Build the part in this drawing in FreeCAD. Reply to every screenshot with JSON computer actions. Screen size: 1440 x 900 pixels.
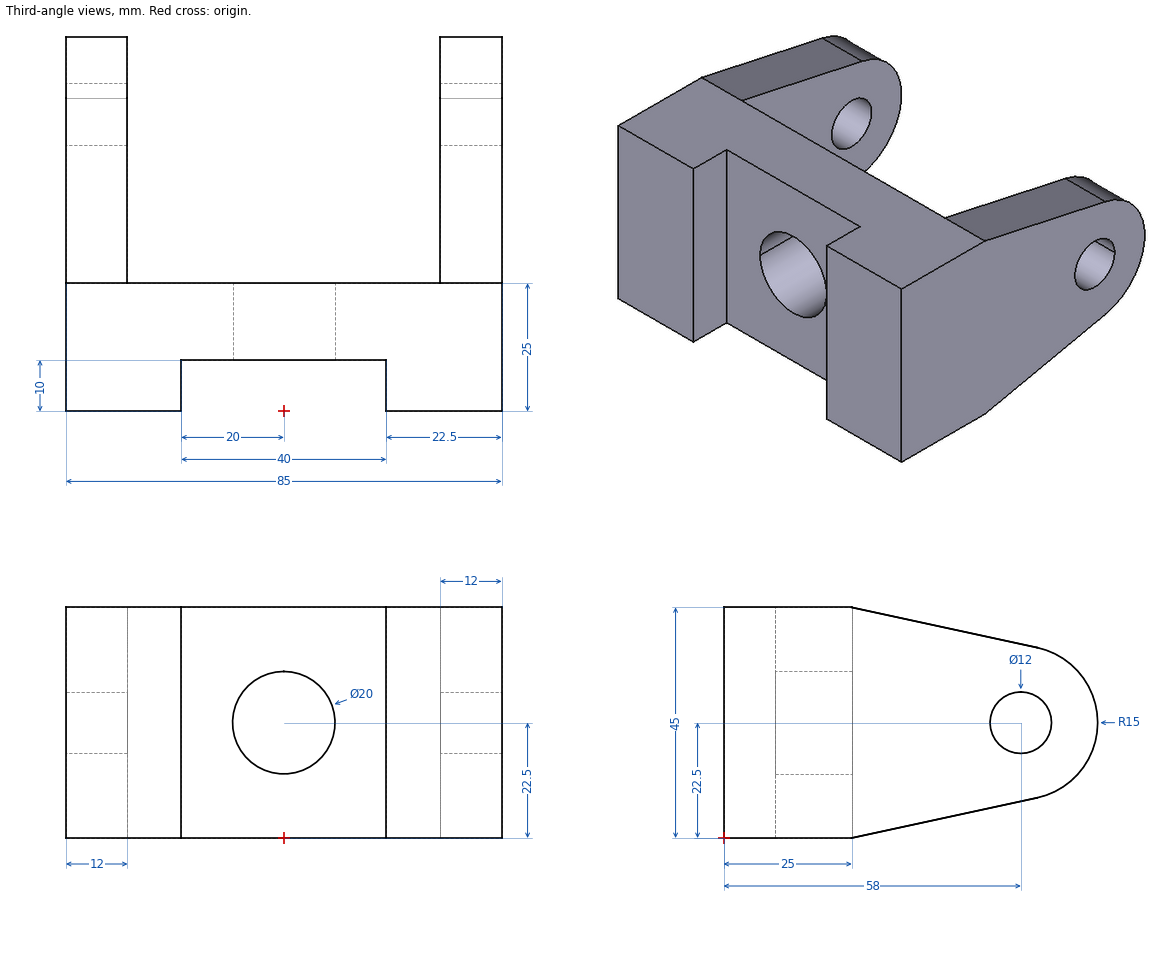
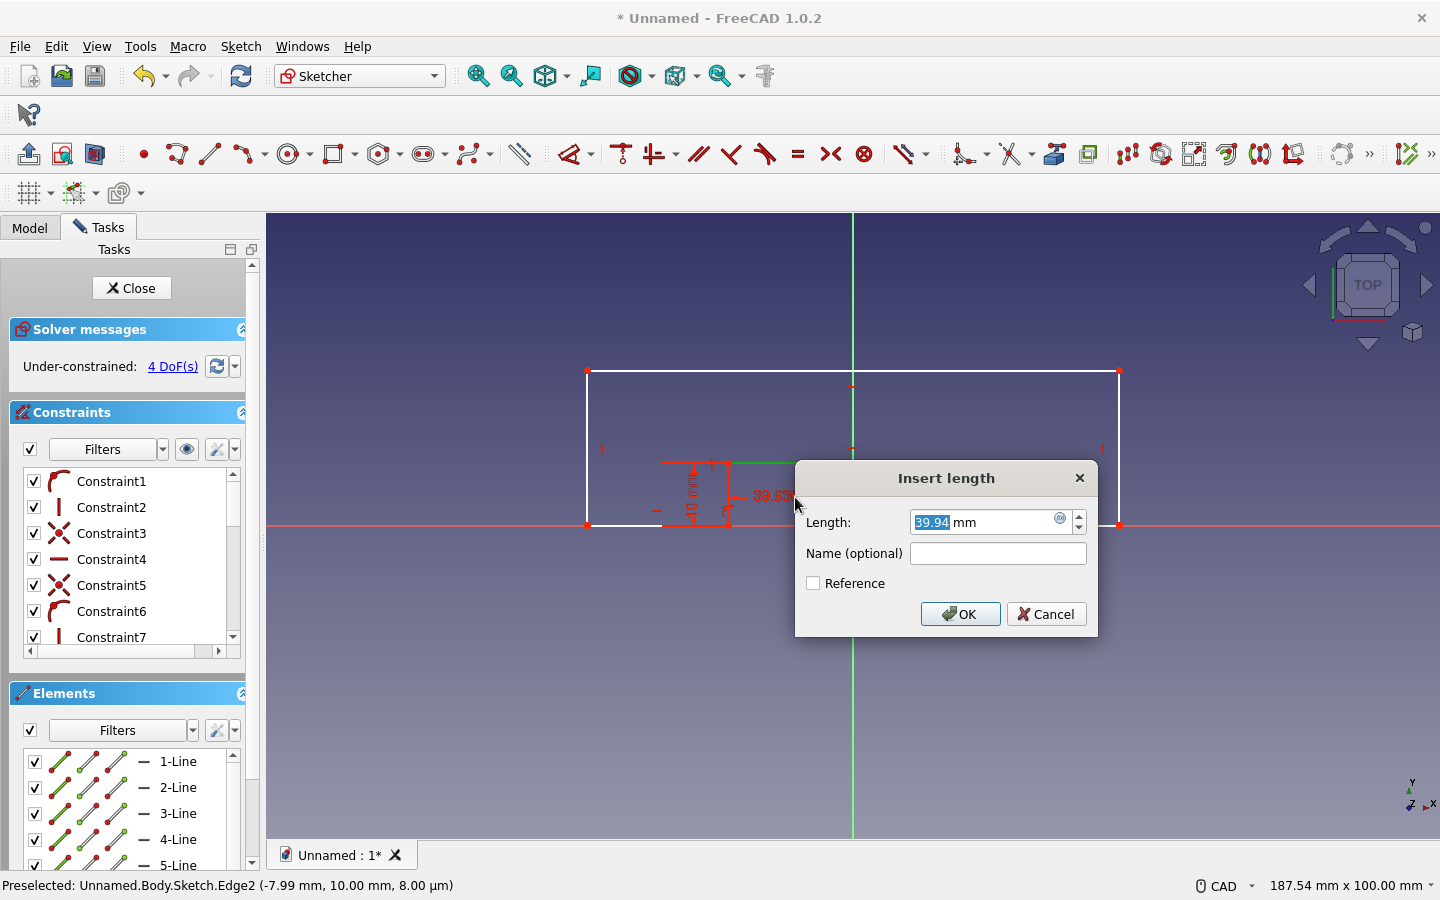
{"action": "type", "text": "40"}
{"action": "key", "text": "Return"}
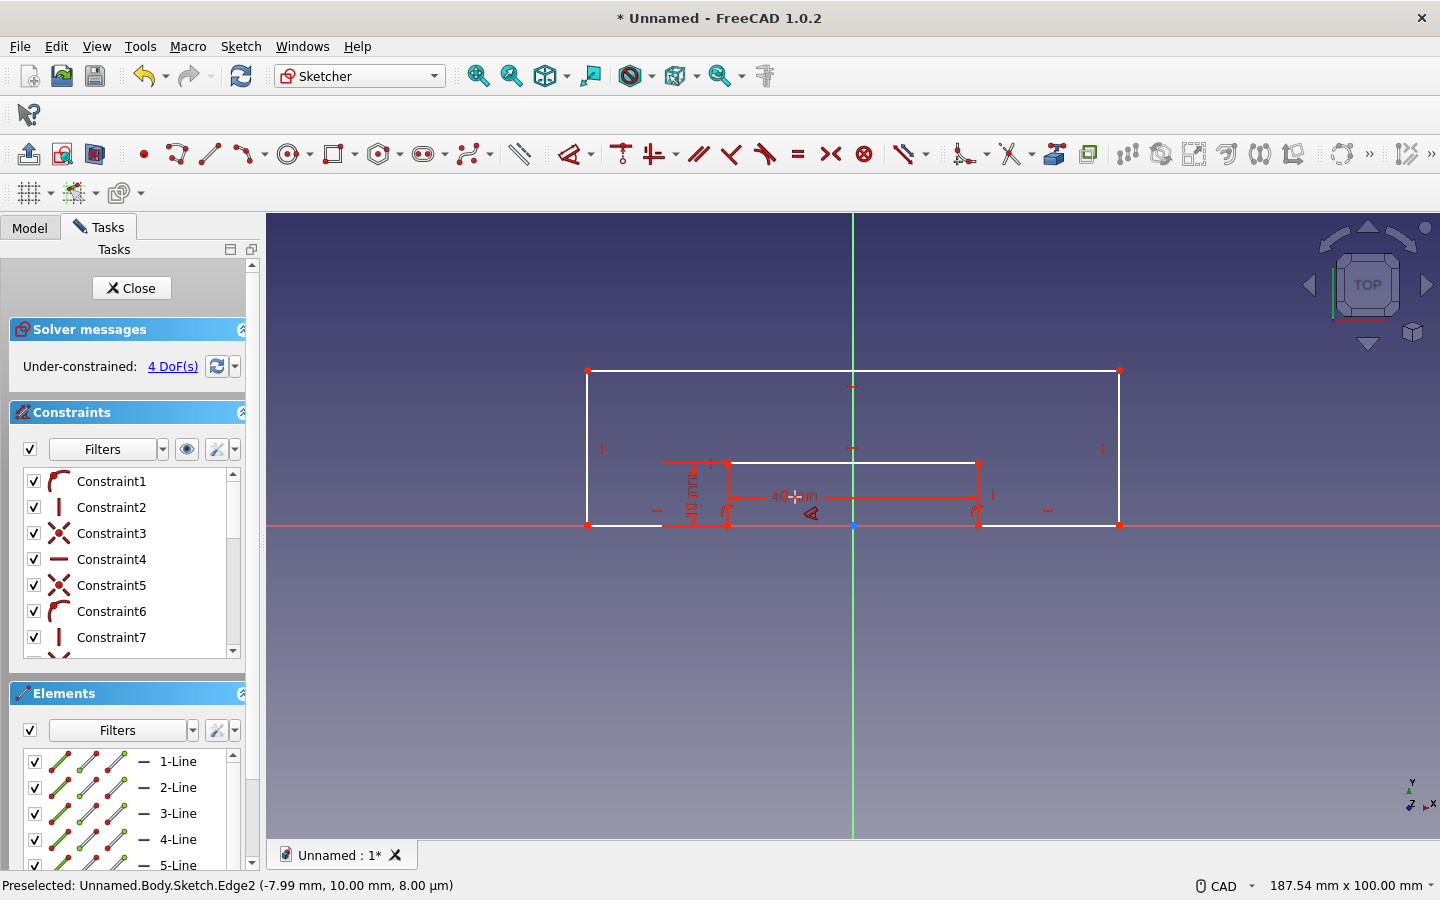
{"action": "left_click", "coordinate": [1119, 479]}
{"action": "left_click", "coordinate": [1153, 448]}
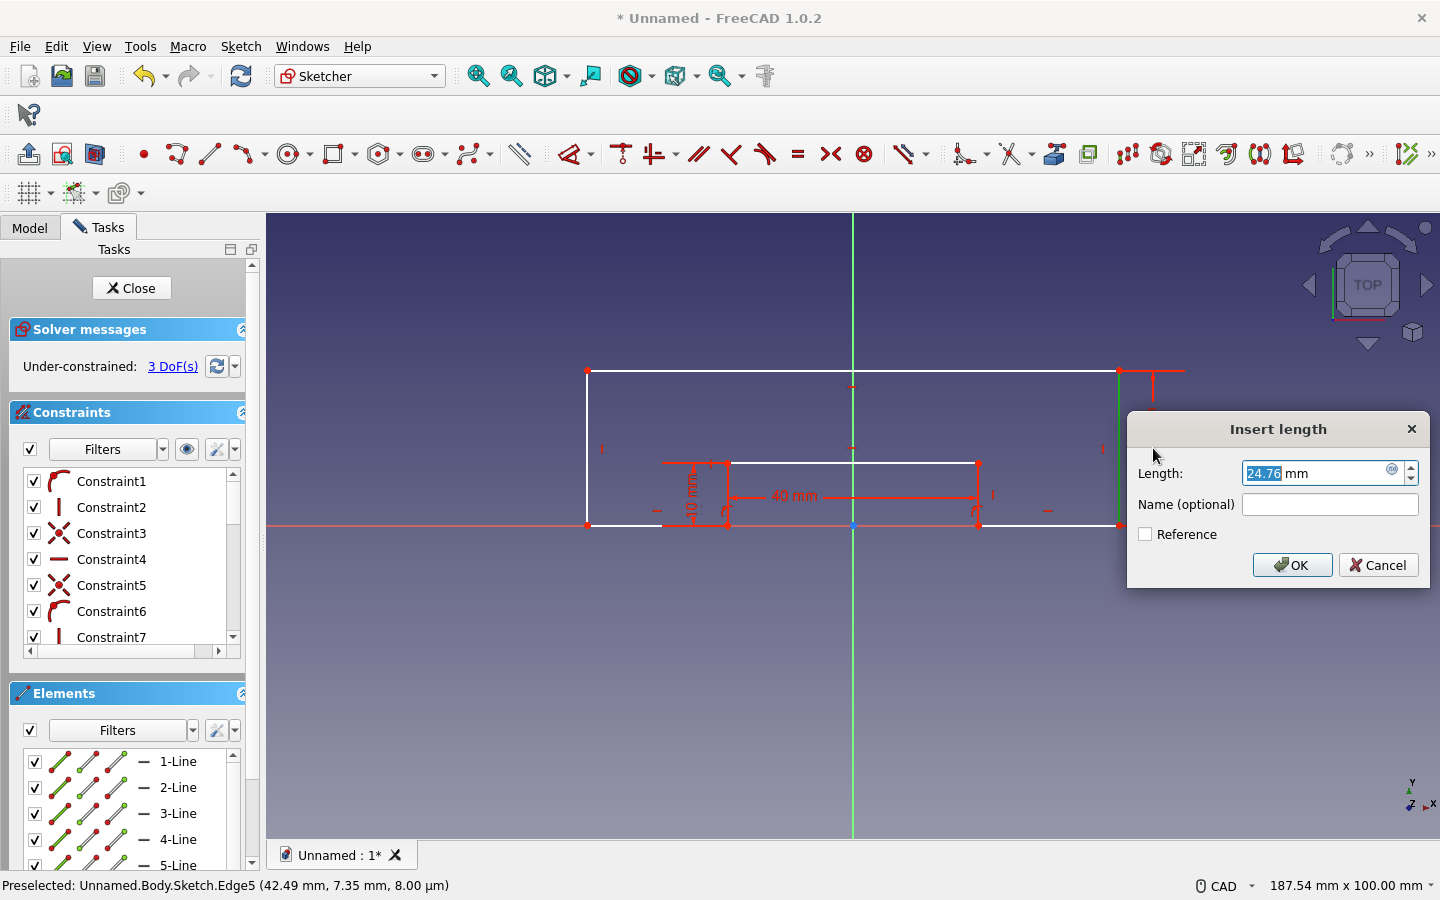
{"action": "type", "text": "25"}
{"action": "key", "text": "Return"}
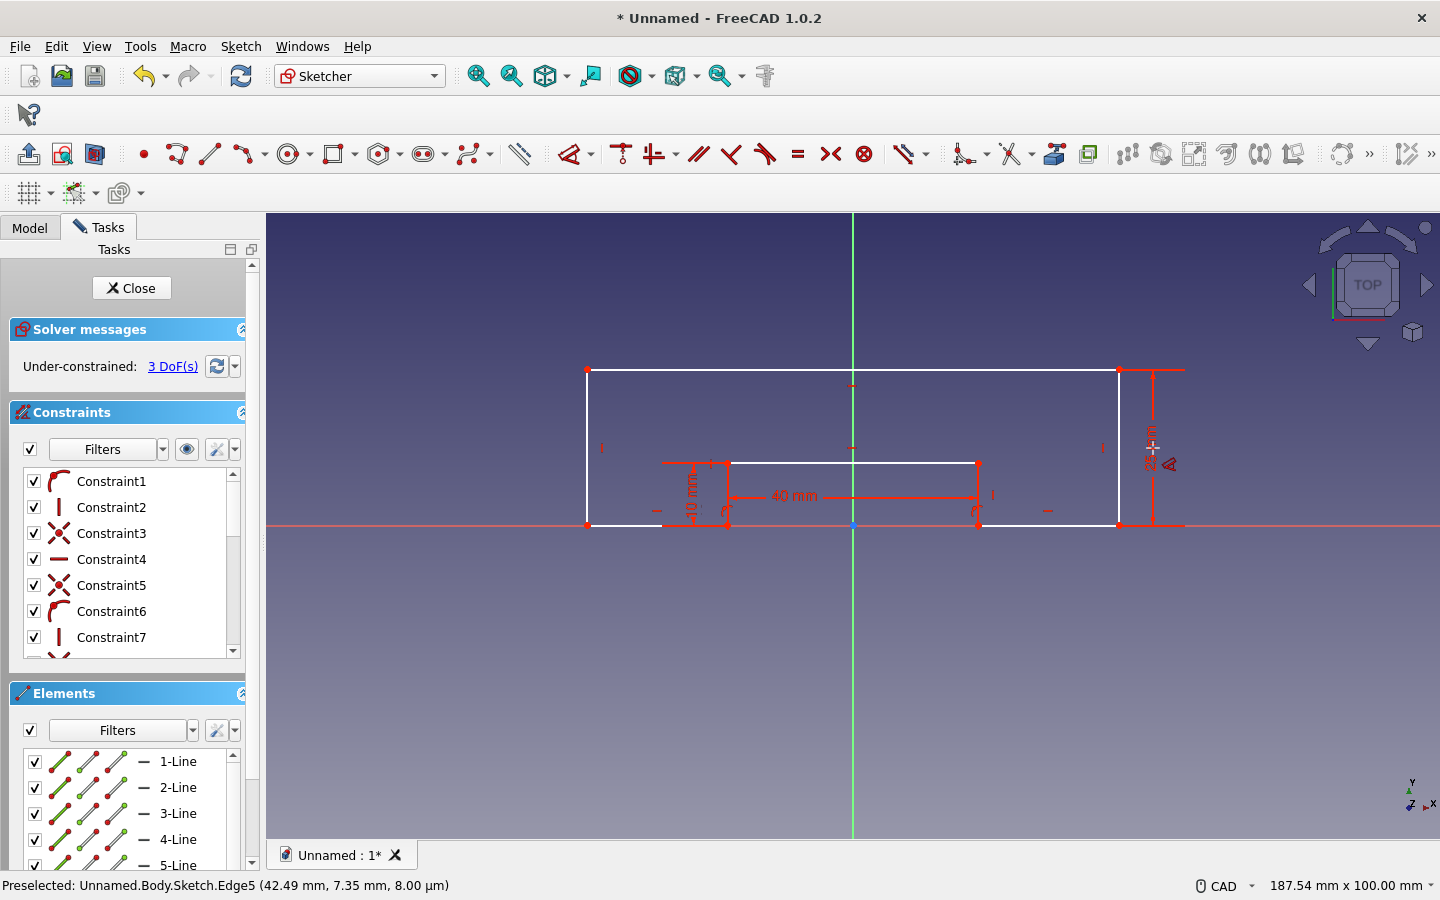
{"action": "left_click", "coordinate": [959, 370]}
{"action": "left_click", "coordinate": [731, 336]}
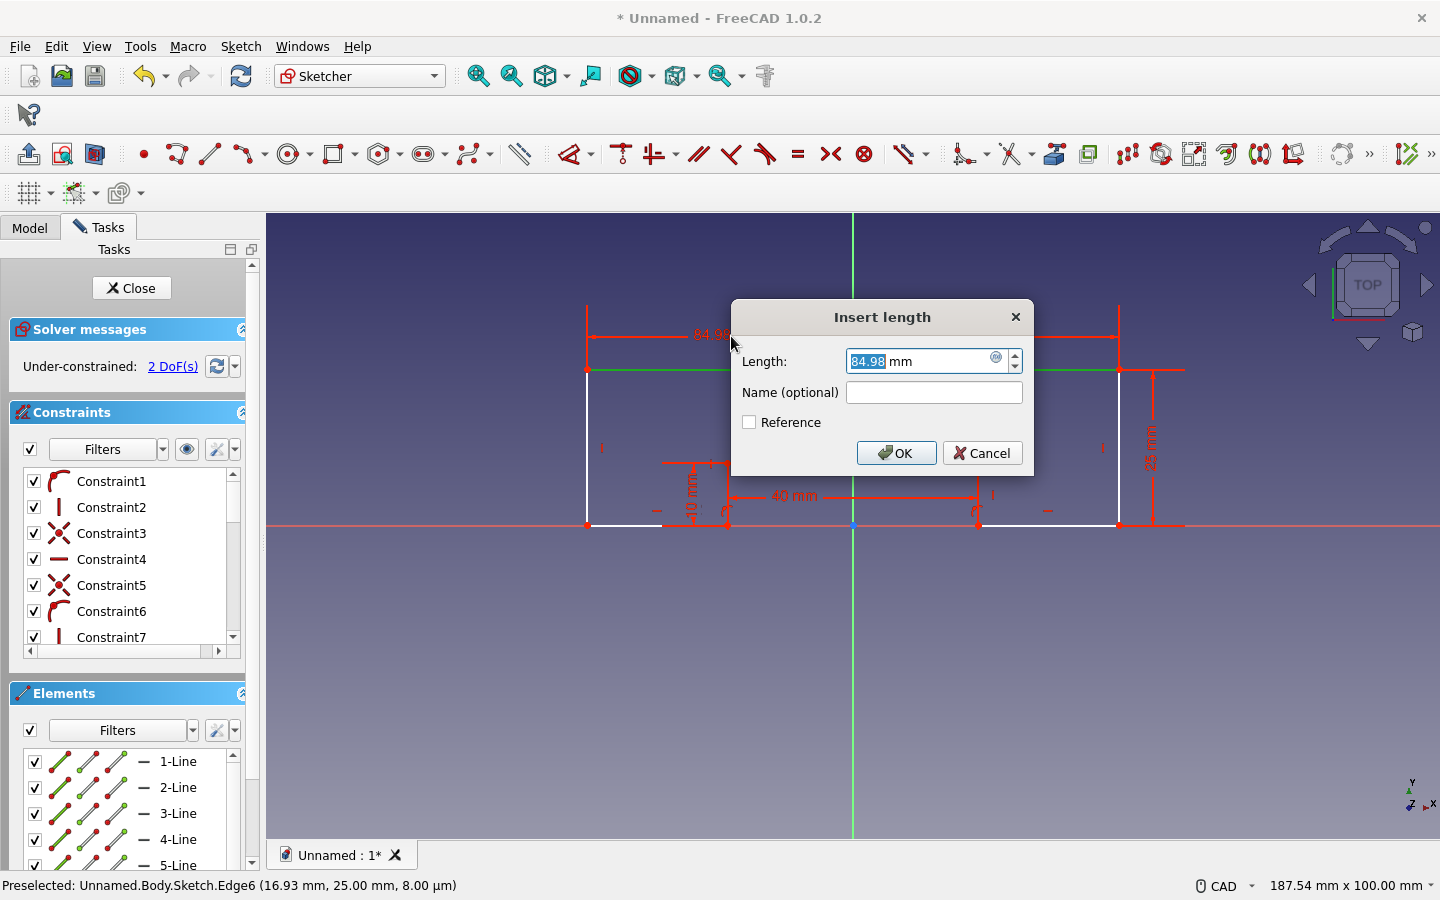
{"action": "type", "text": "85"}
{"action": "key", "text": "Return"}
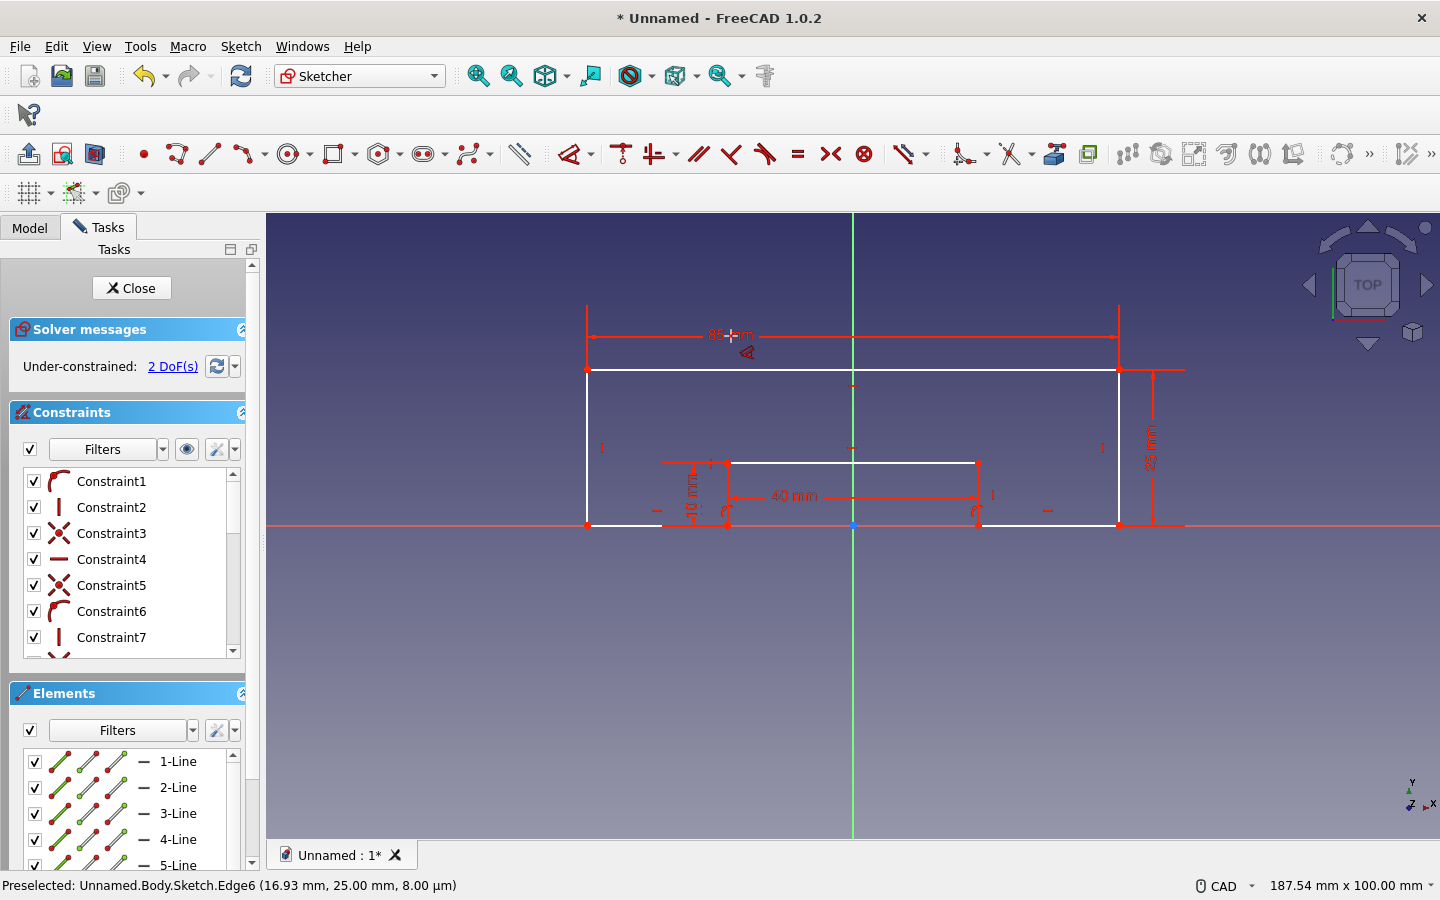
{"action": "left_click", "coordinate": [728, 526]}
{"action": "left_click", "coordinate": [790, 560]}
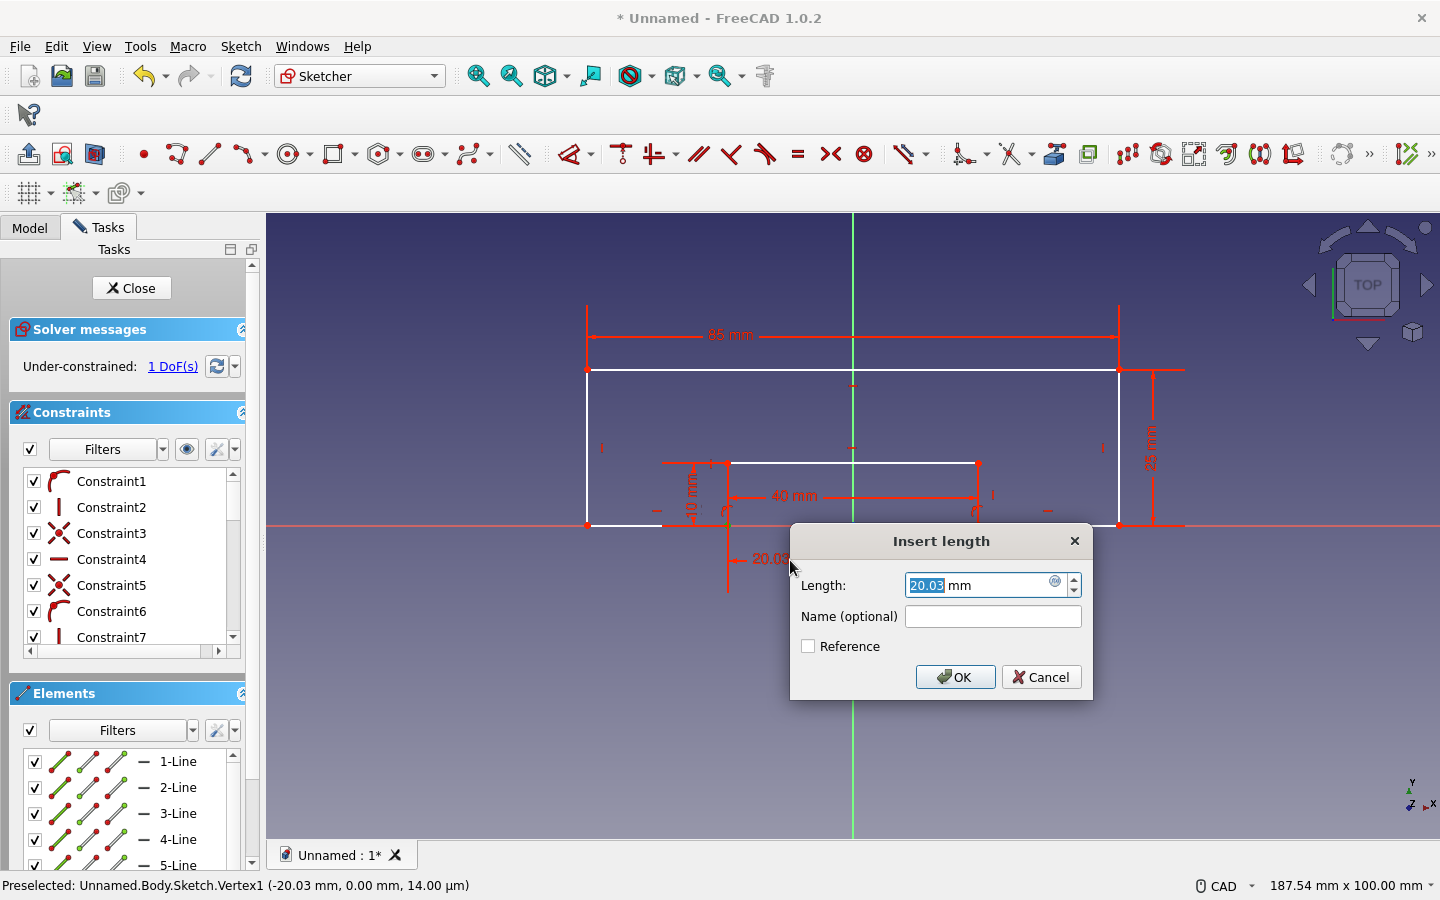
{"action": "type", "text": "20"}
{"action": "key", "text": "Return"}